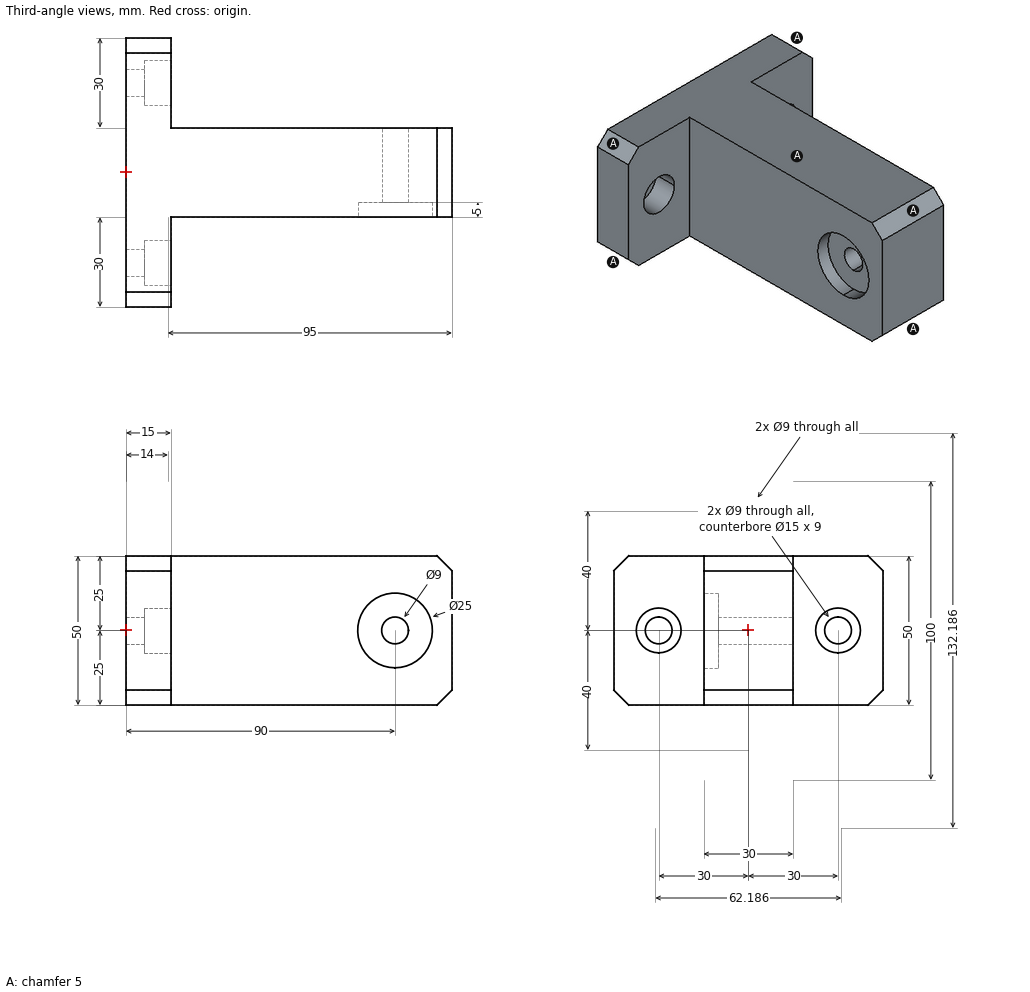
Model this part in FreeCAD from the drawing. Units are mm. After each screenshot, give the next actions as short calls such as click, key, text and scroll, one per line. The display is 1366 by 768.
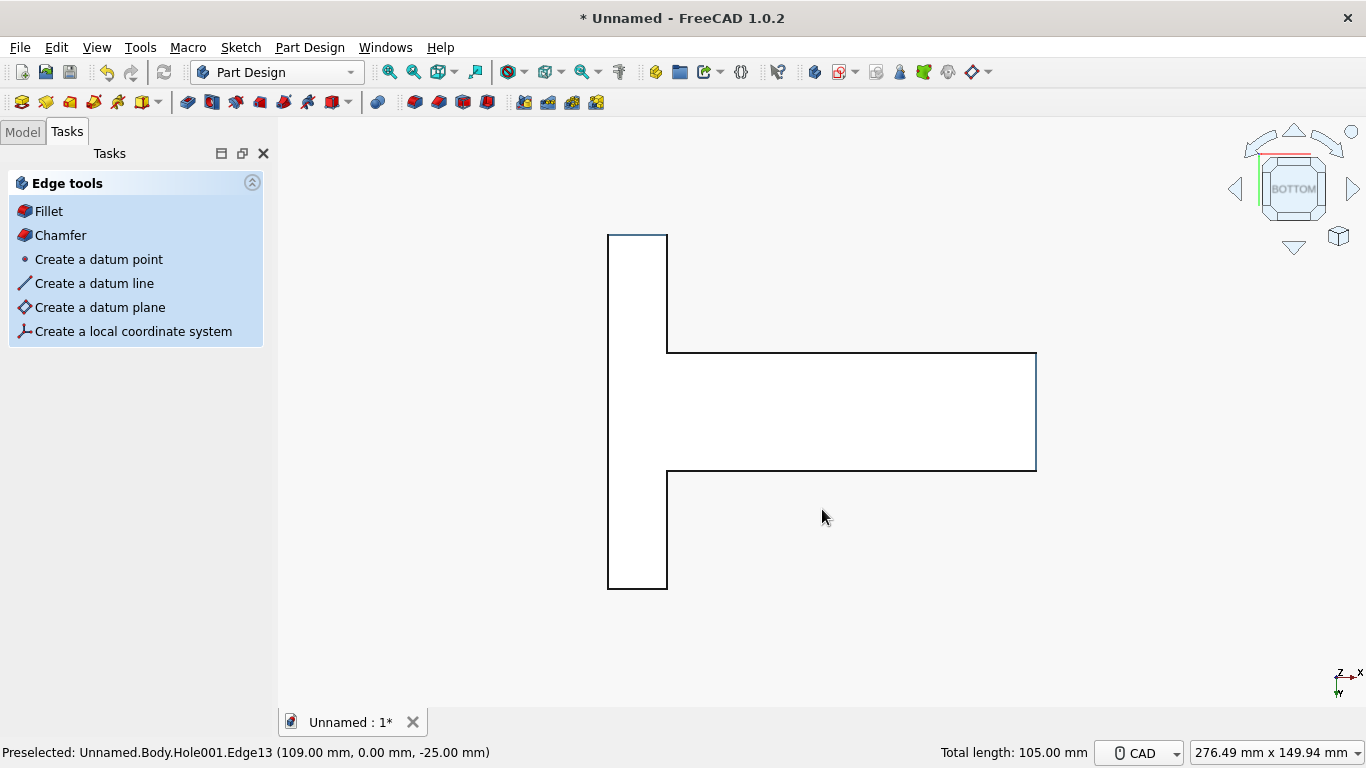
click(637, 588, ctrl)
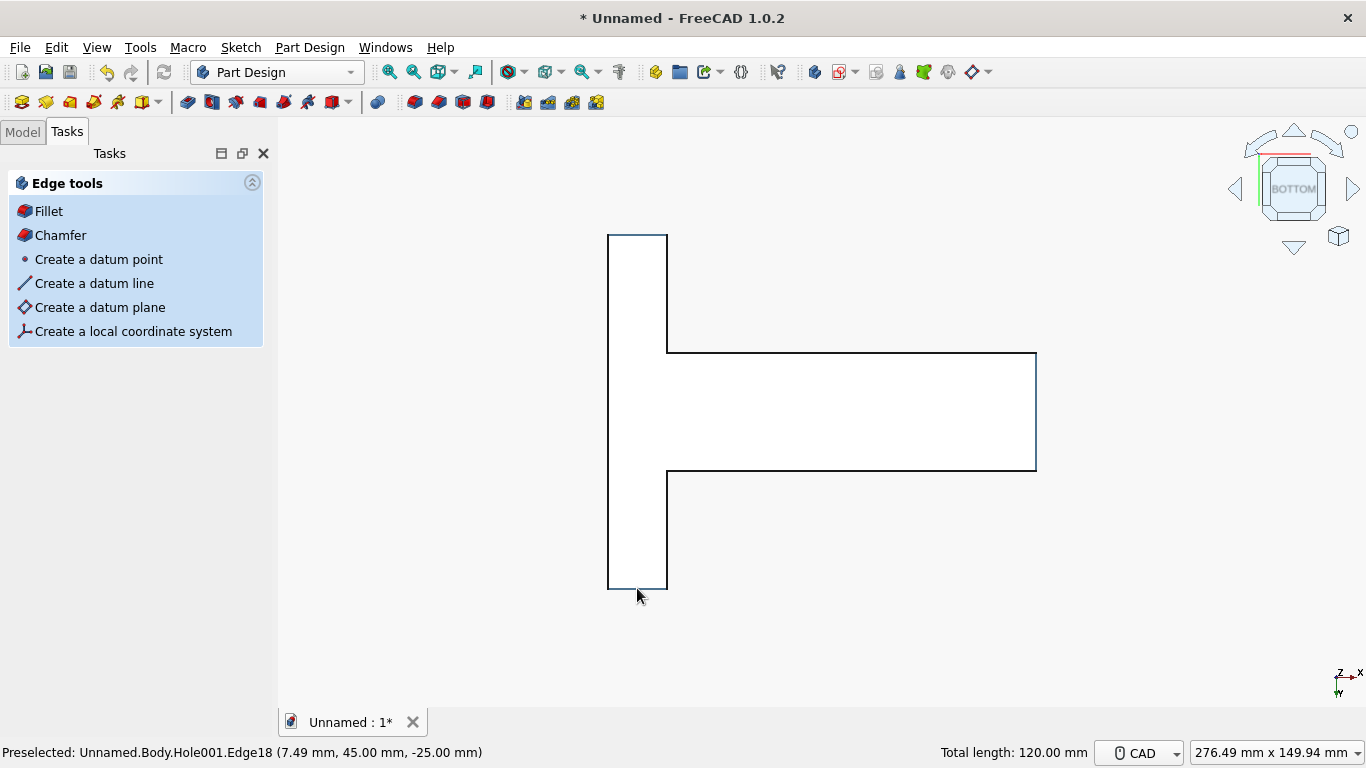
click(440, 102)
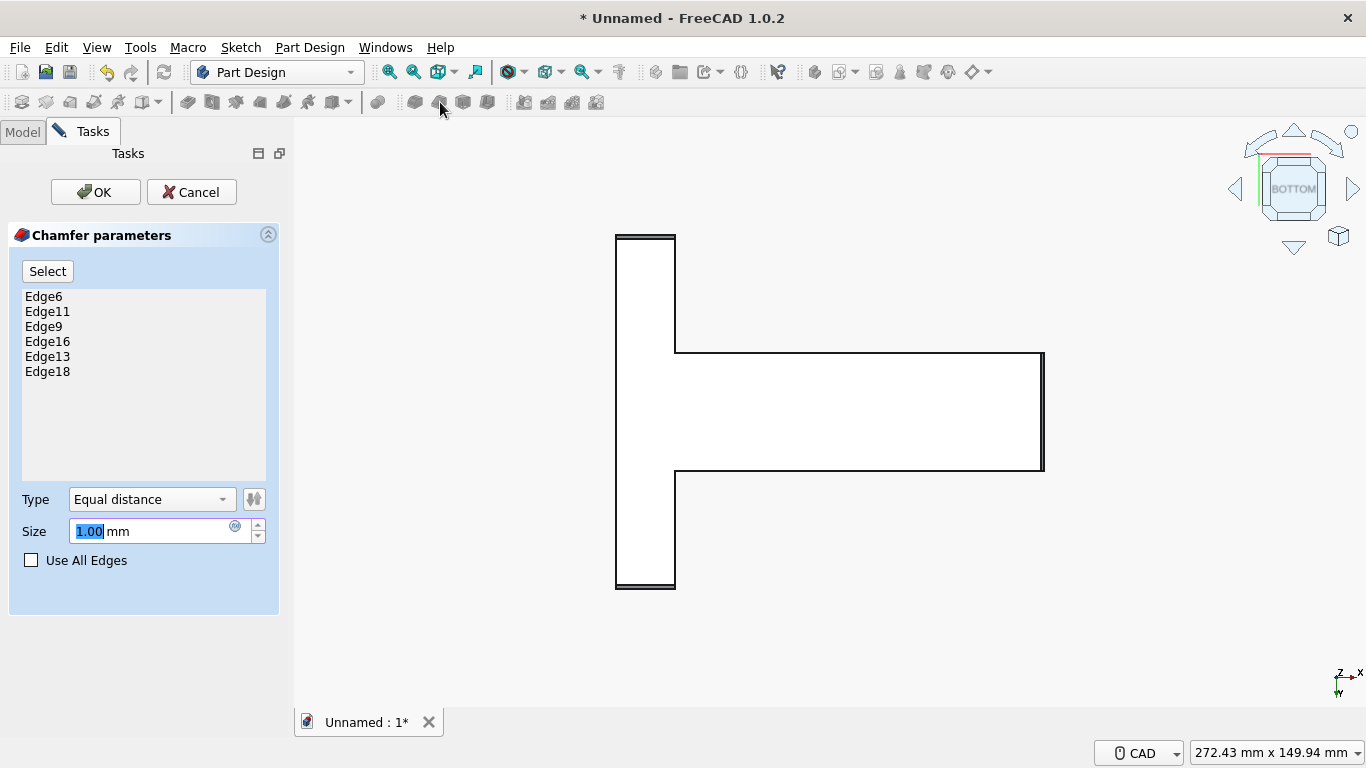
text(5)
key(Tab)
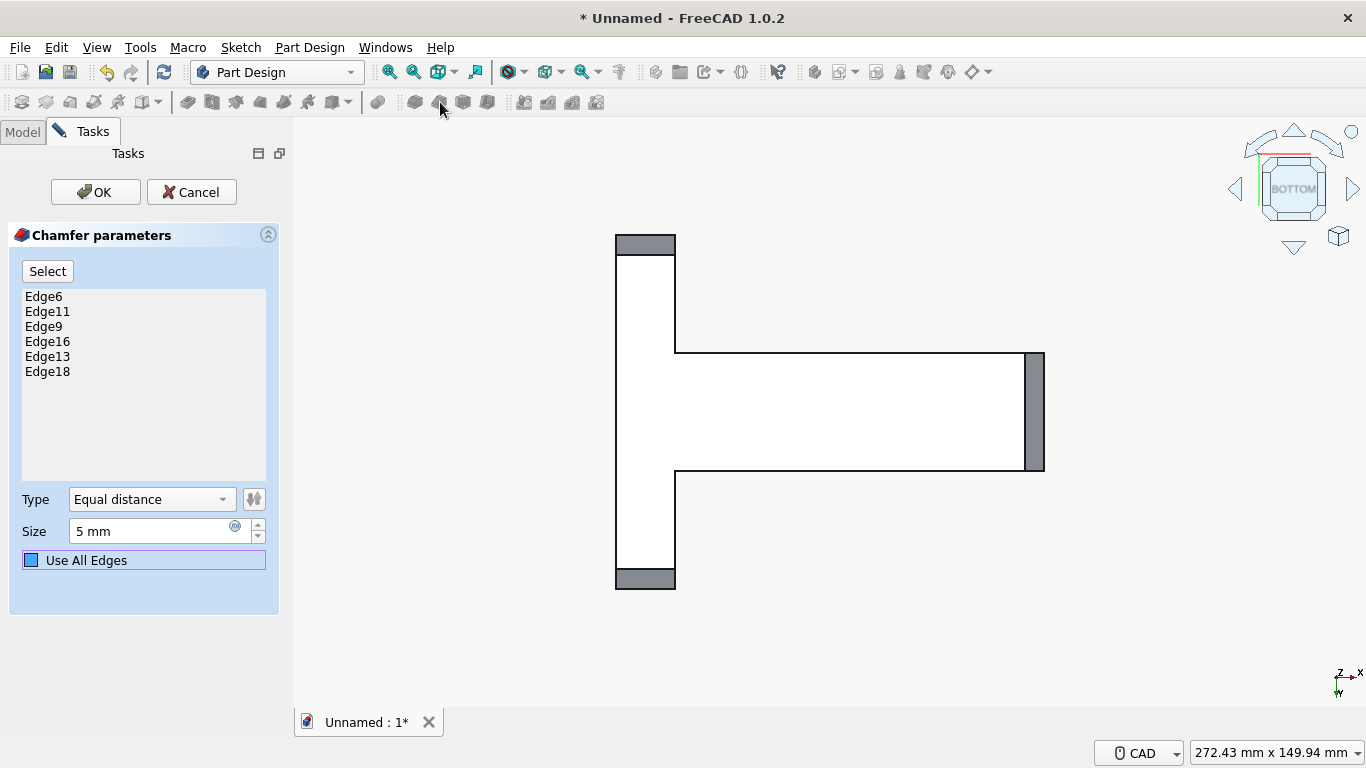
click(96, 192)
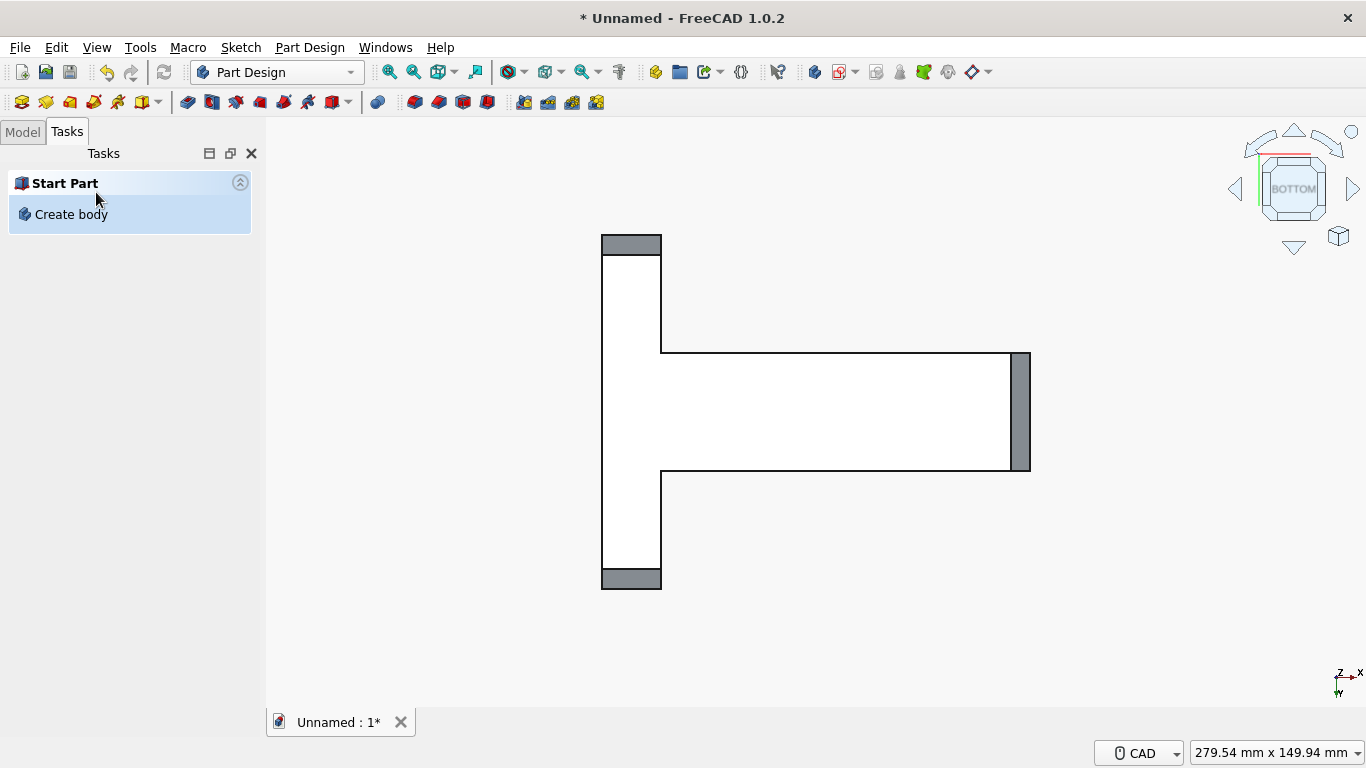
key(0)